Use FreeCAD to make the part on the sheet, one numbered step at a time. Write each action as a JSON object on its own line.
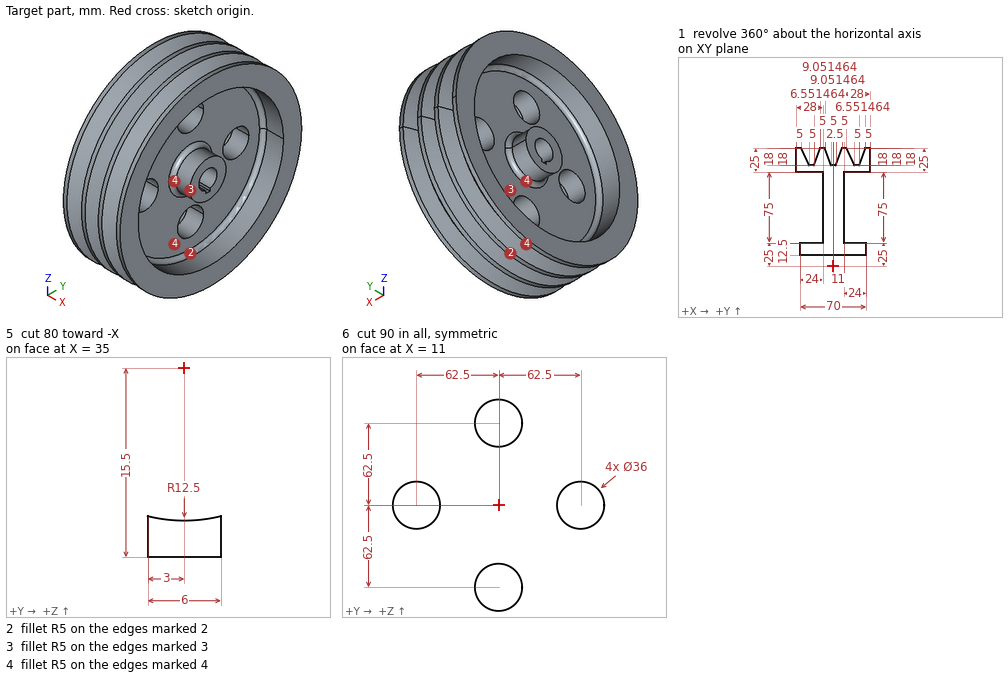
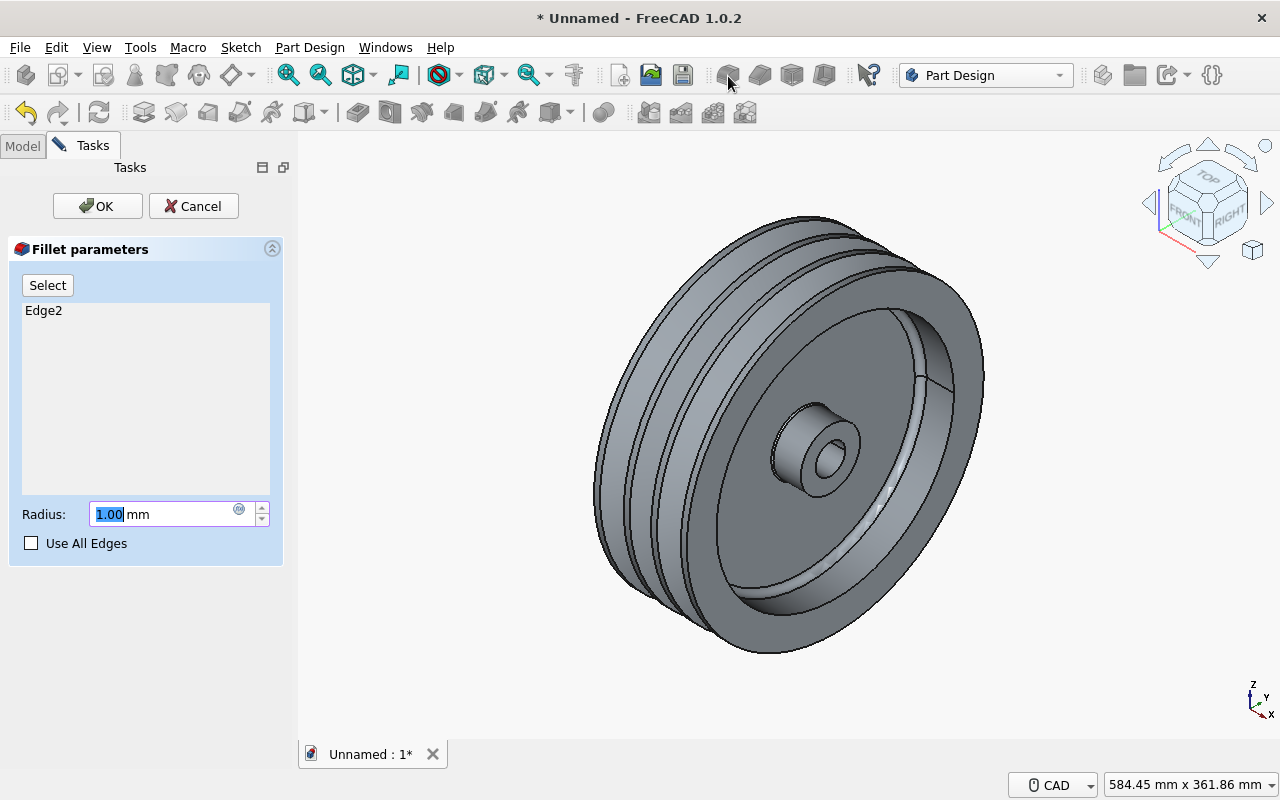
{"action": "type", "text": "5"}
{"action": "key", "text": "Tab"}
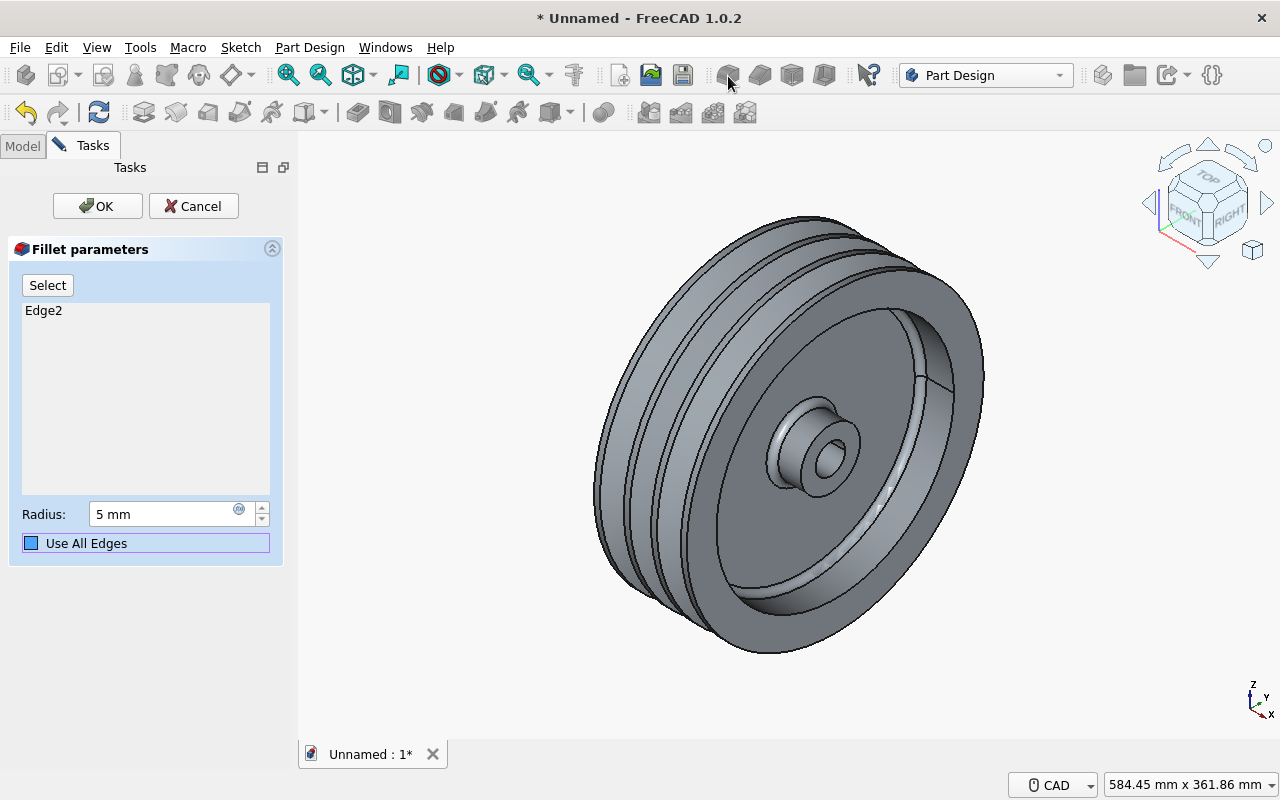
{"action": "left_click", "coordinate": [98, 206]}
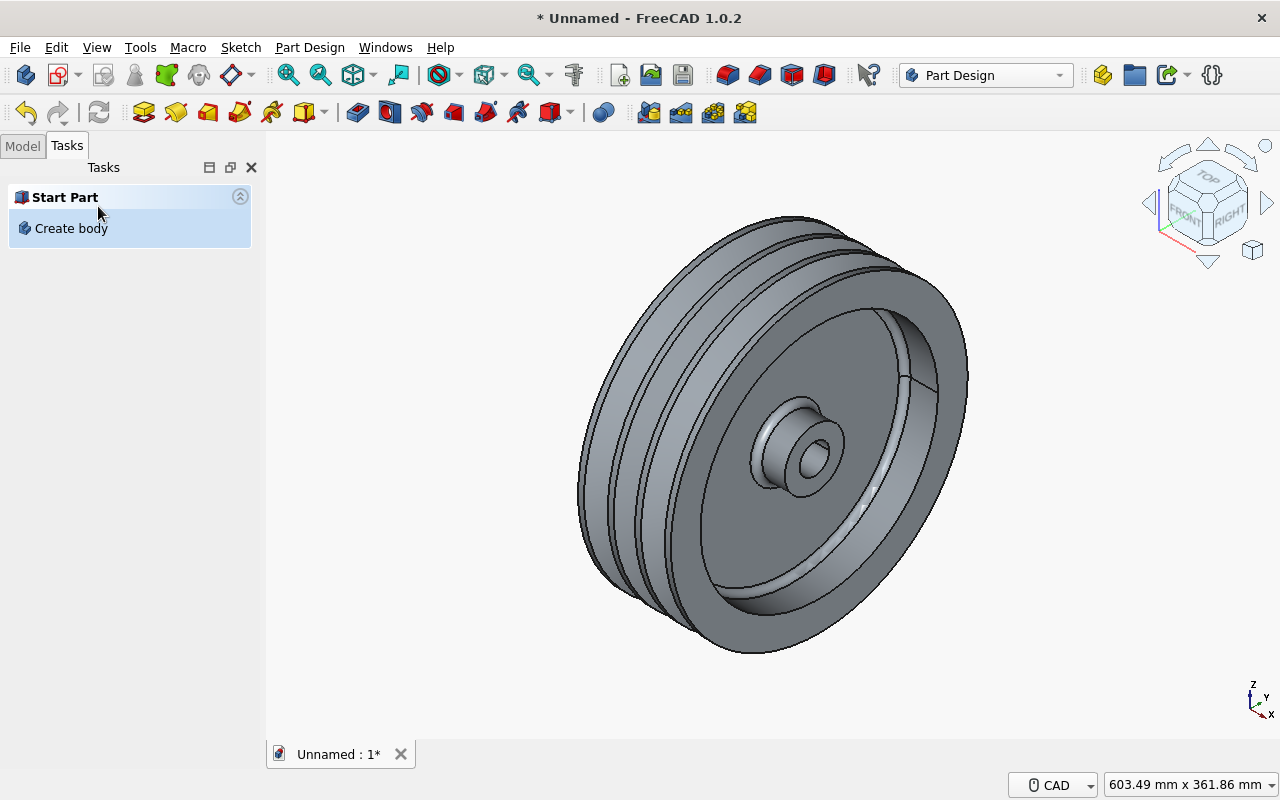
{"action": "key", "text": "2"}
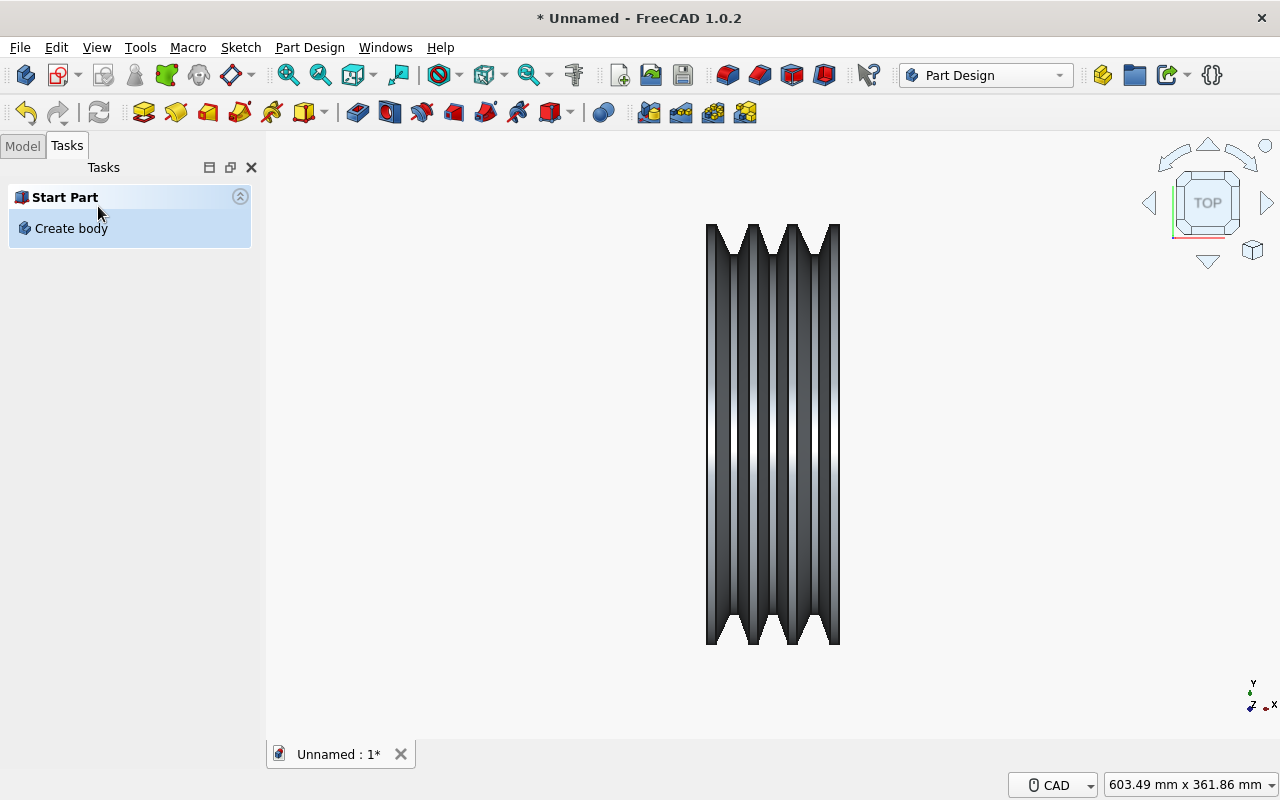
{"action": "key", "text": "0"}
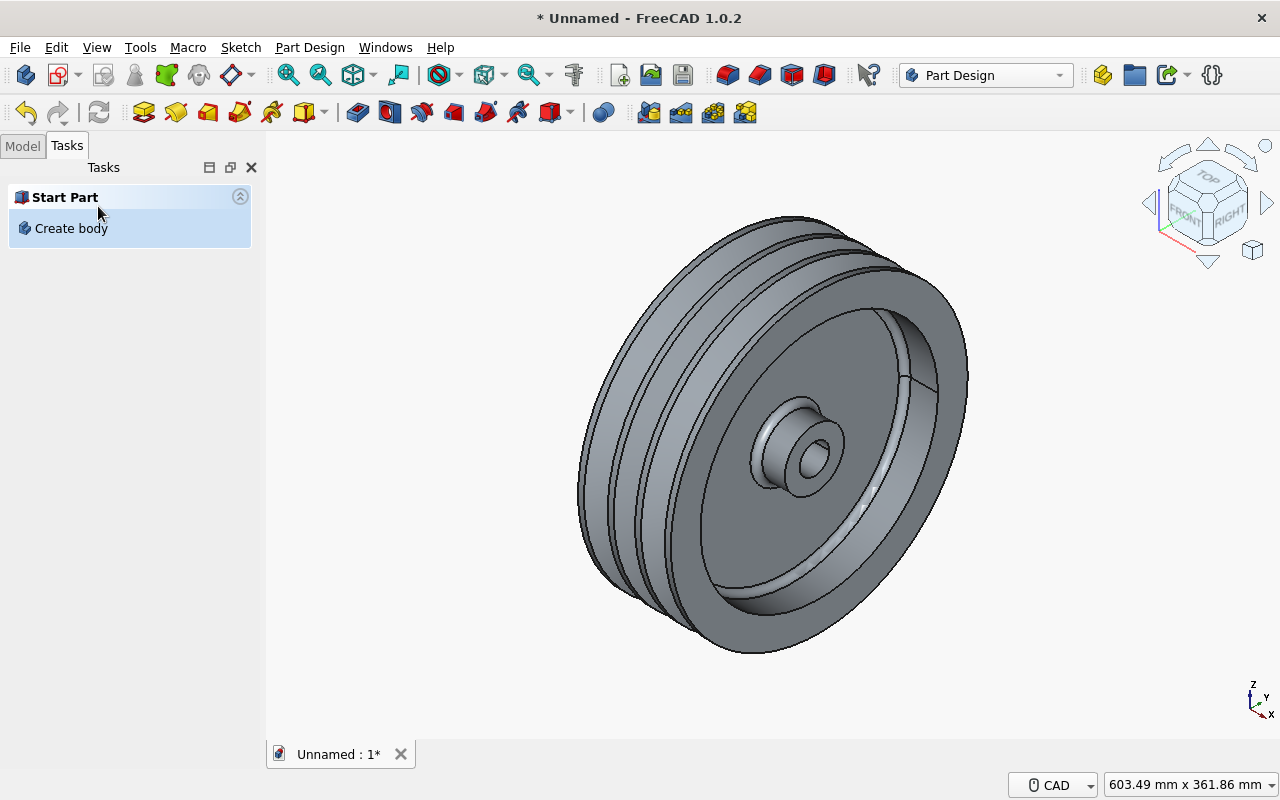
{"action": "key", "text": "1"}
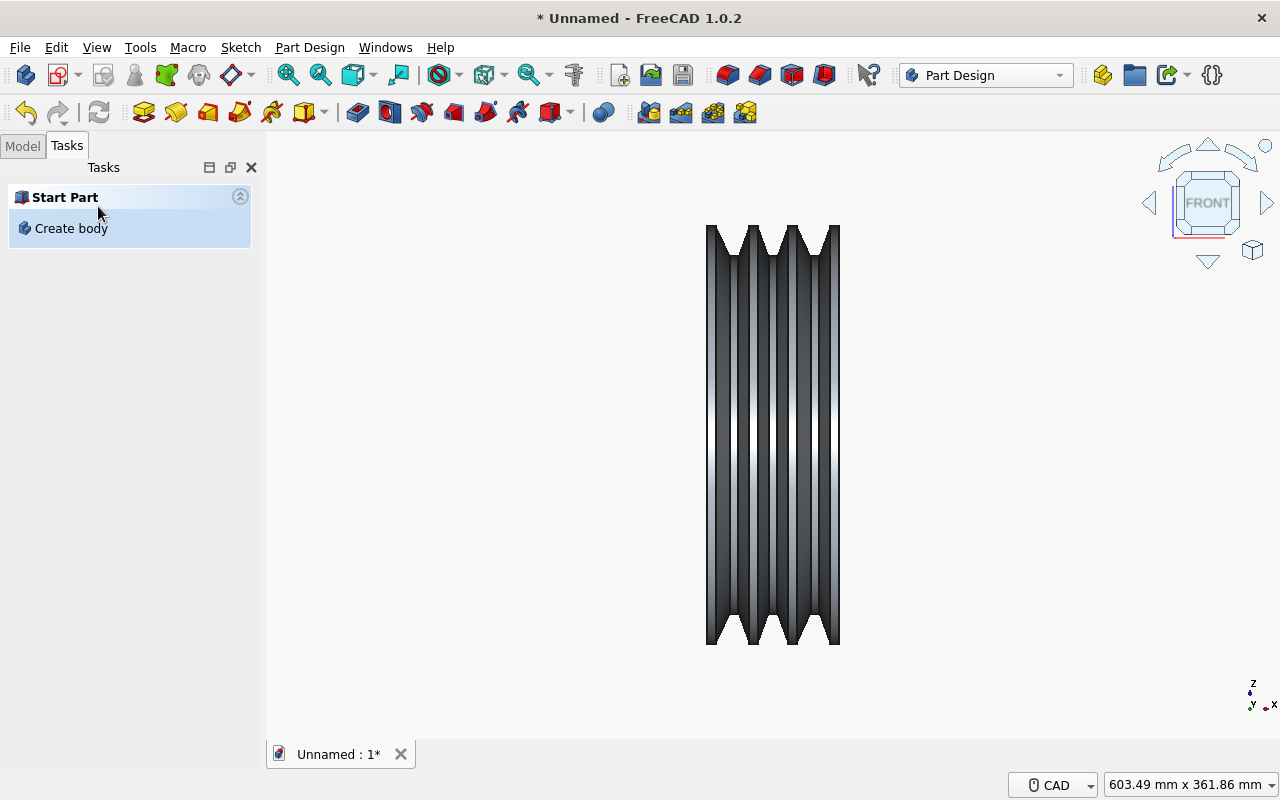
{"action": "key", "text": "3"}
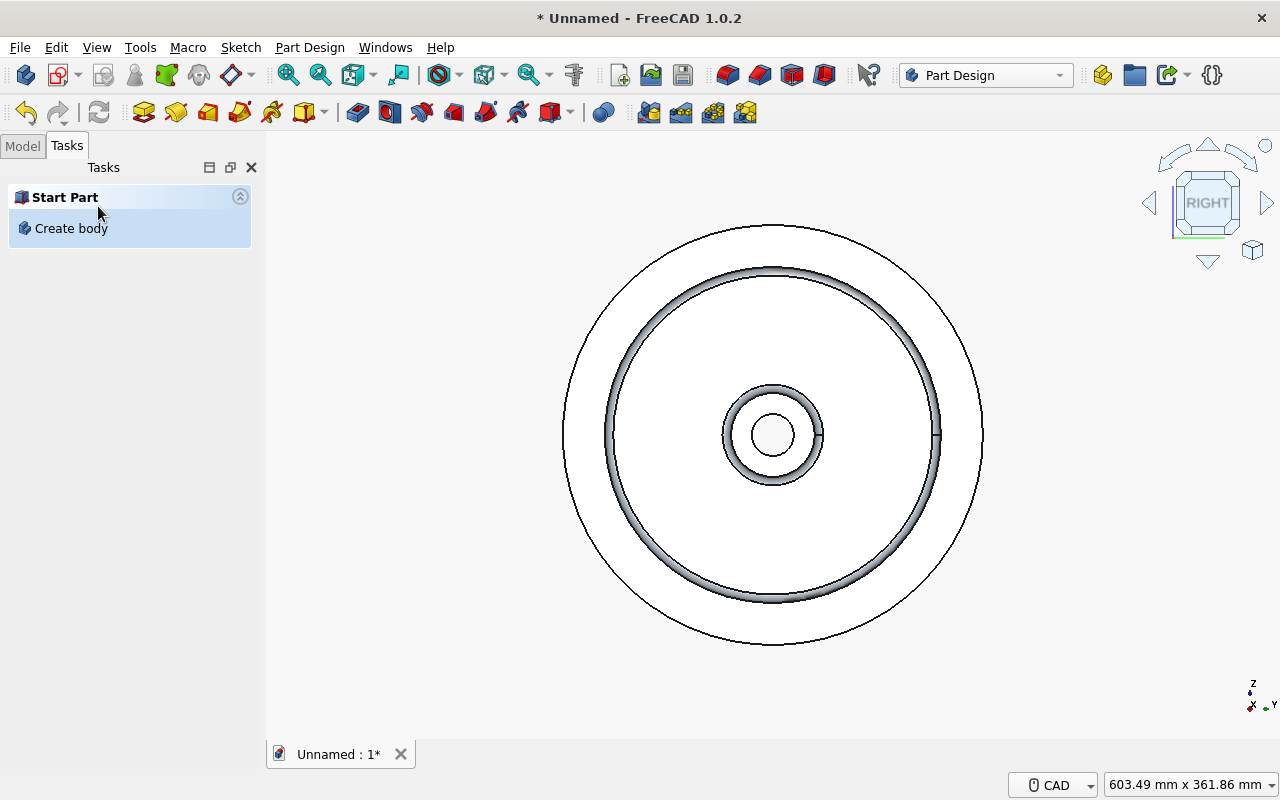
{"action": "key", "text": "5"}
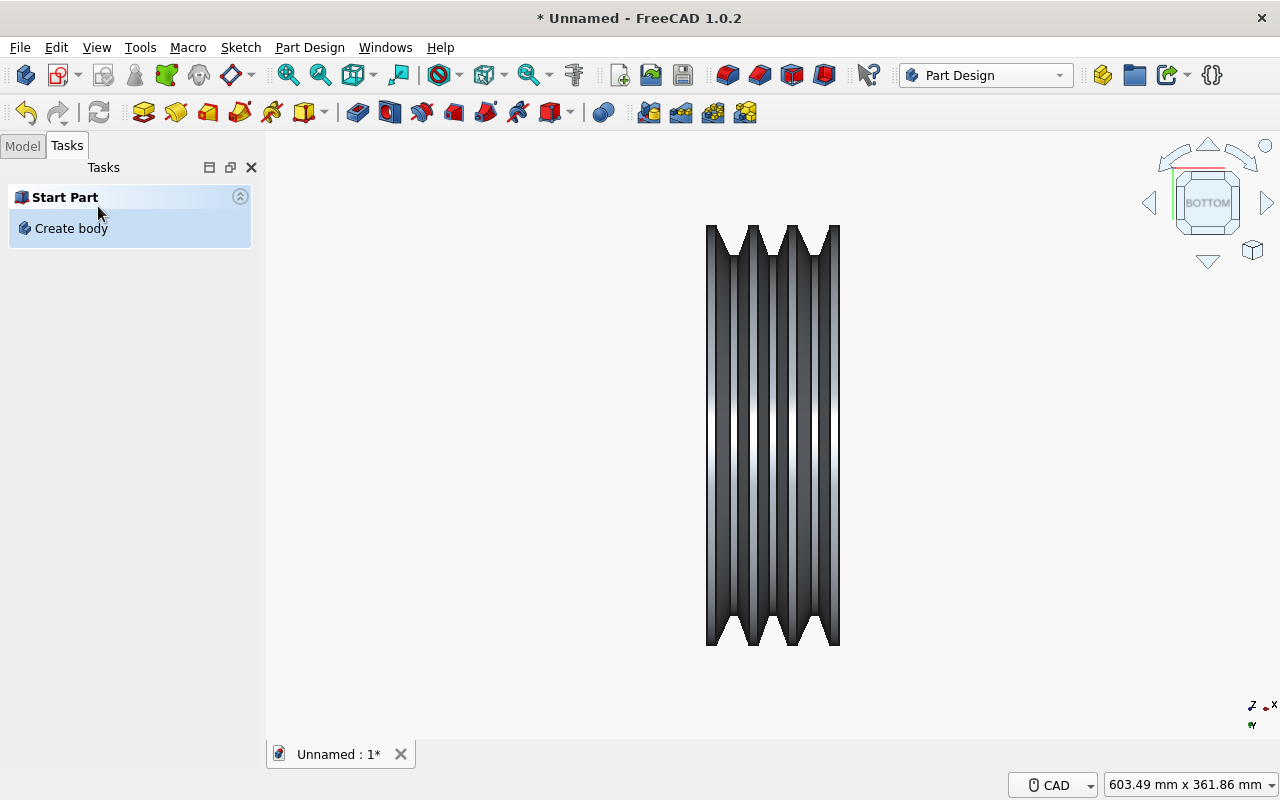
{"action": "key", "text": "4"}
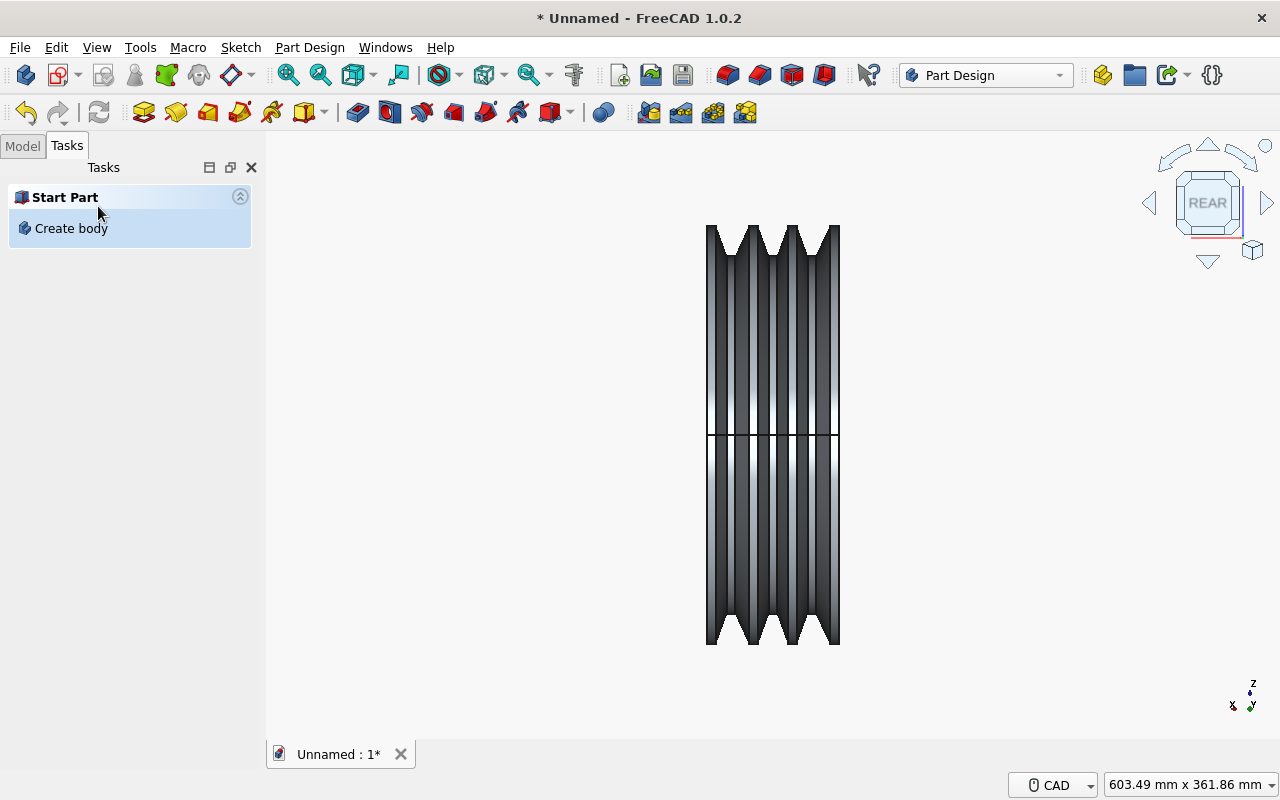
{"action": "key", "text": "6"}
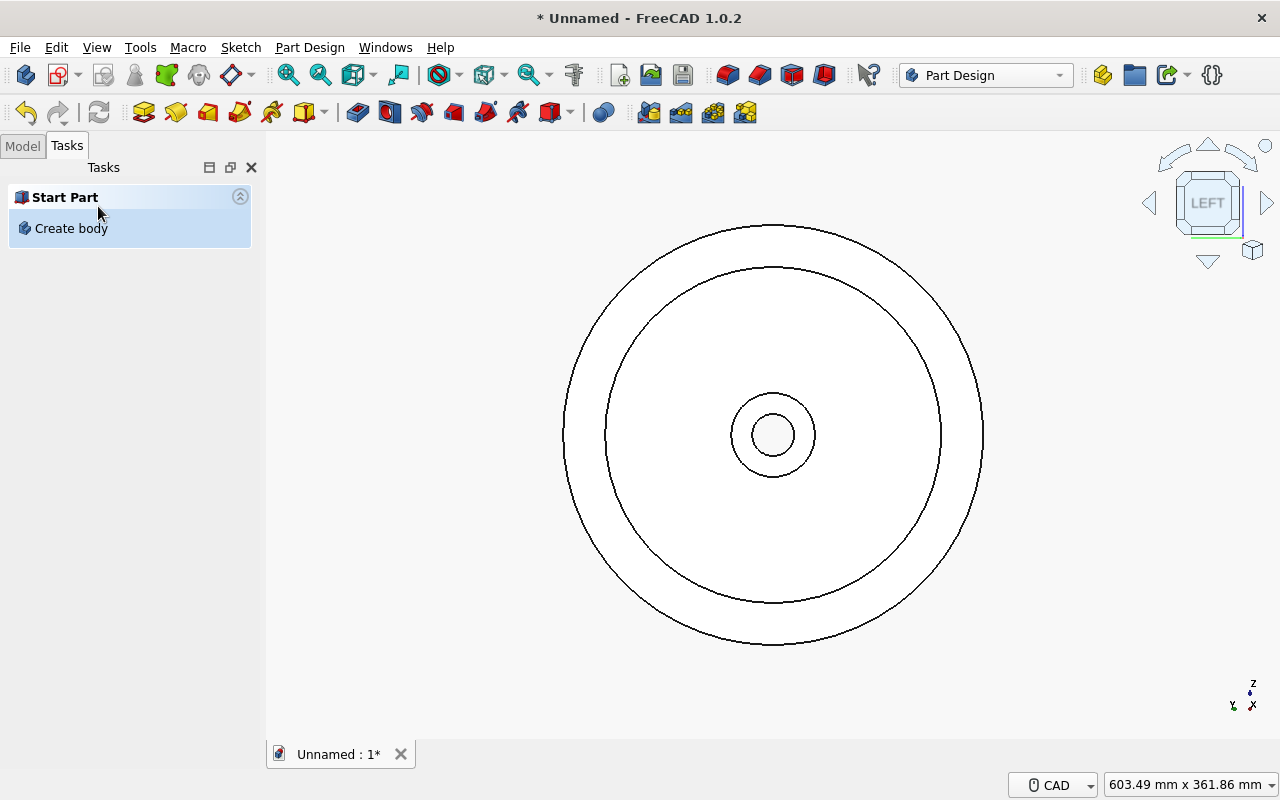
{"action": "key", "text": "v 3"}